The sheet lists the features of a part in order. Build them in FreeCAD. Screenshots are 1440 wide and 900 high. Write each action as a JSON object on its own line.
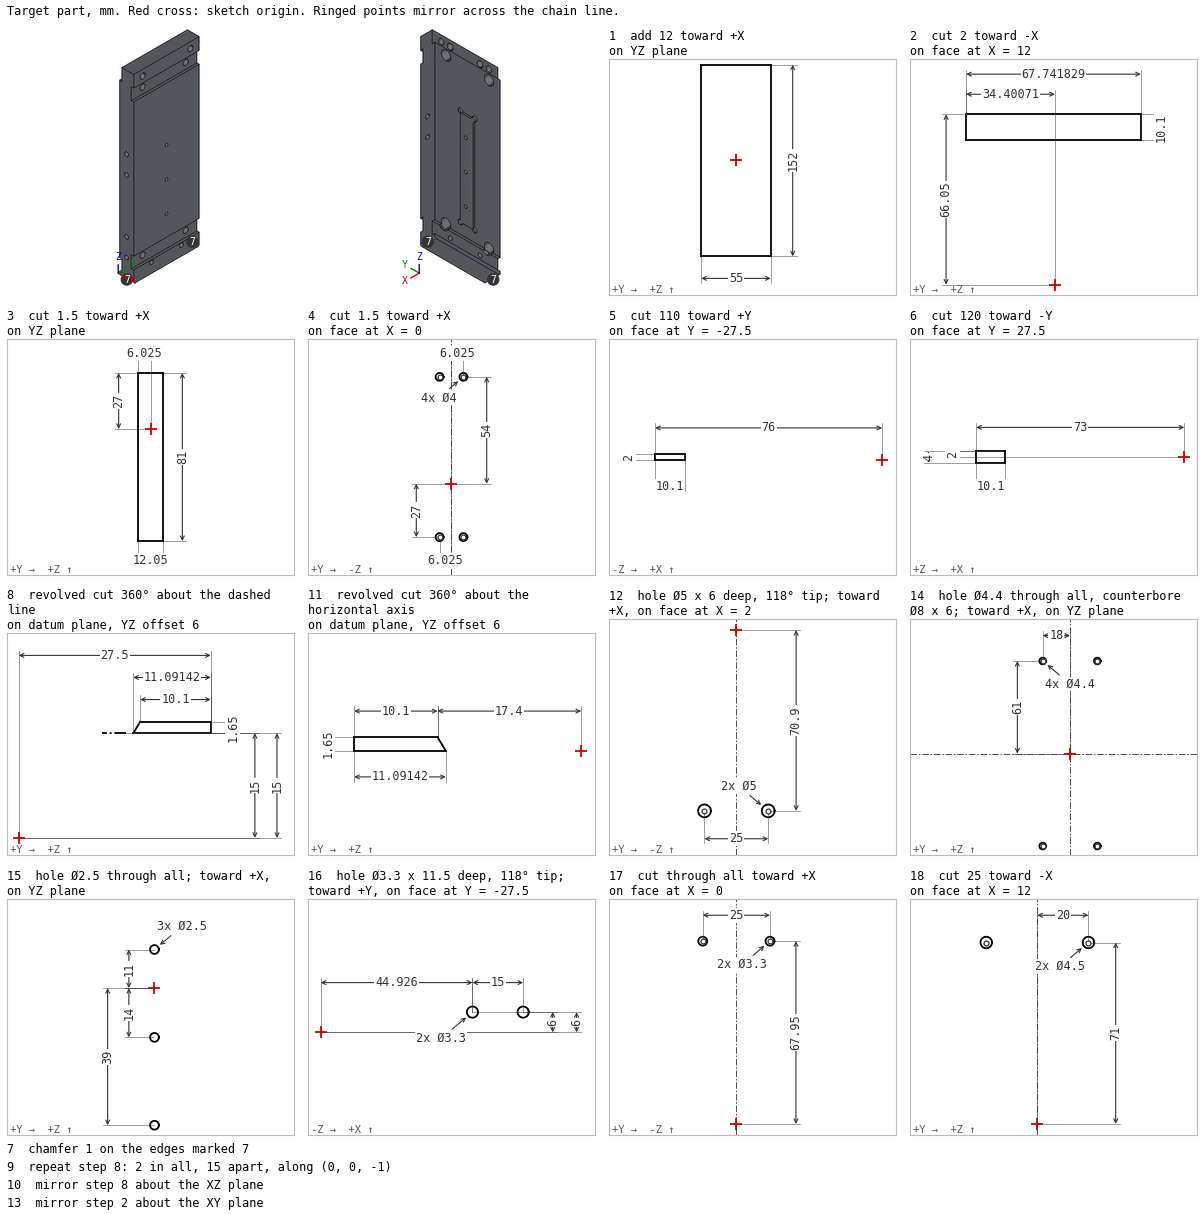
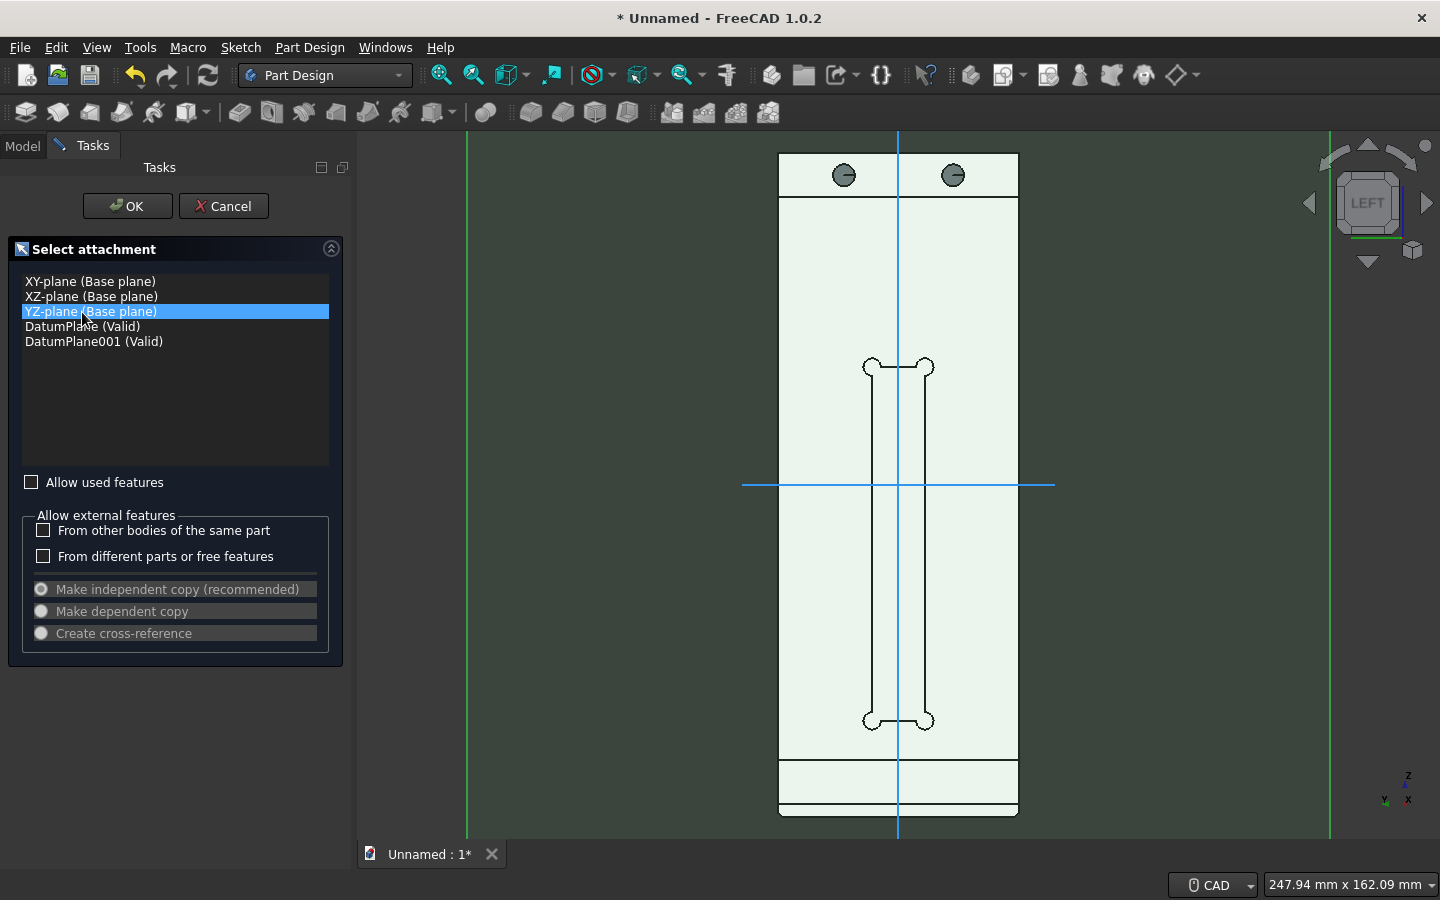
{"action": "left_click", "coordinate": [128, 206]}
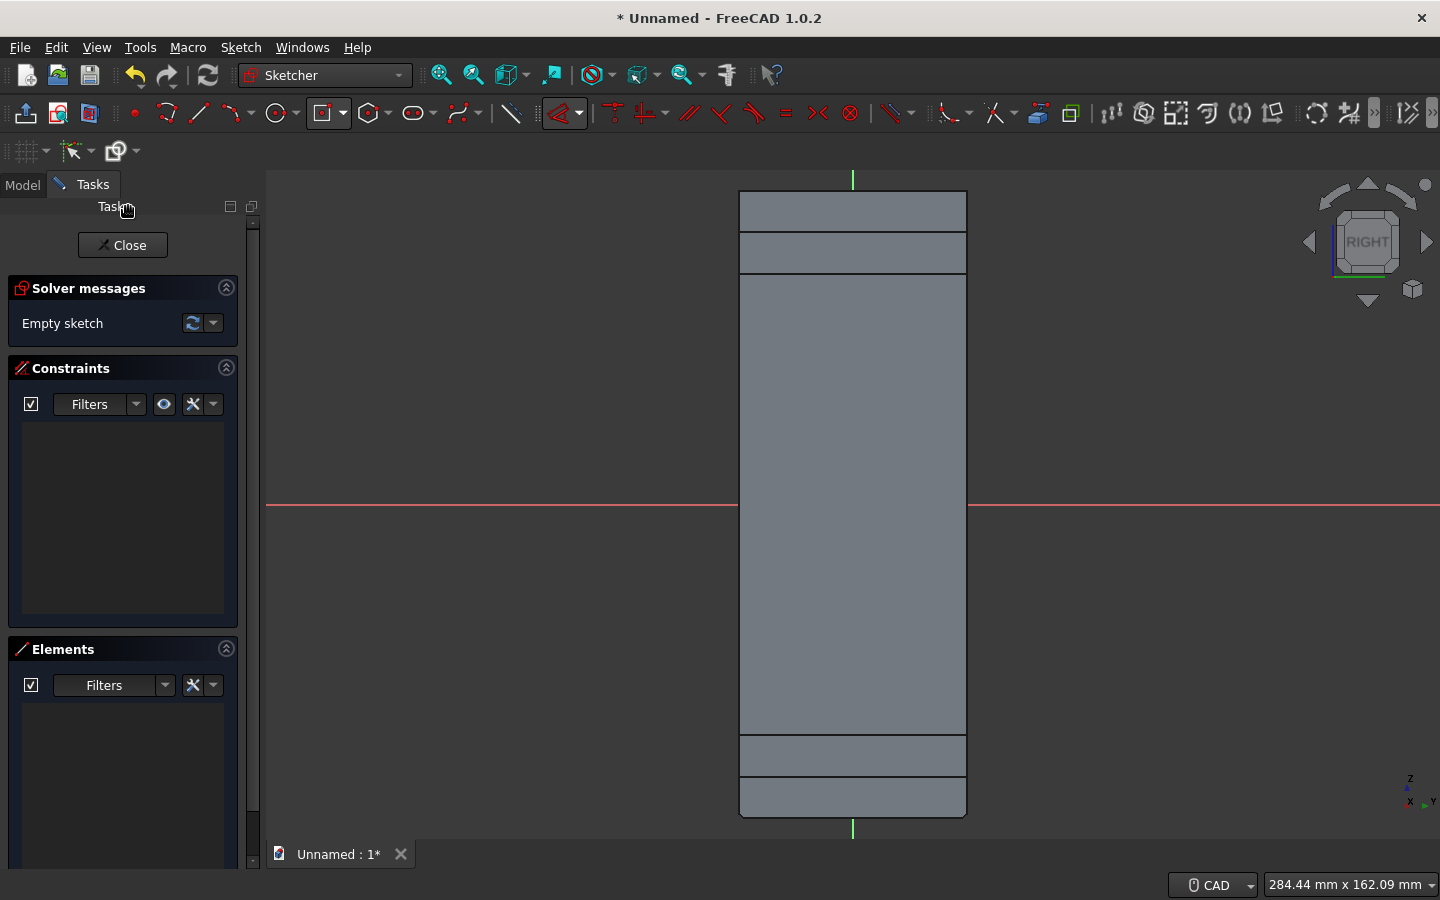
{"action": "key", "text": "q s"}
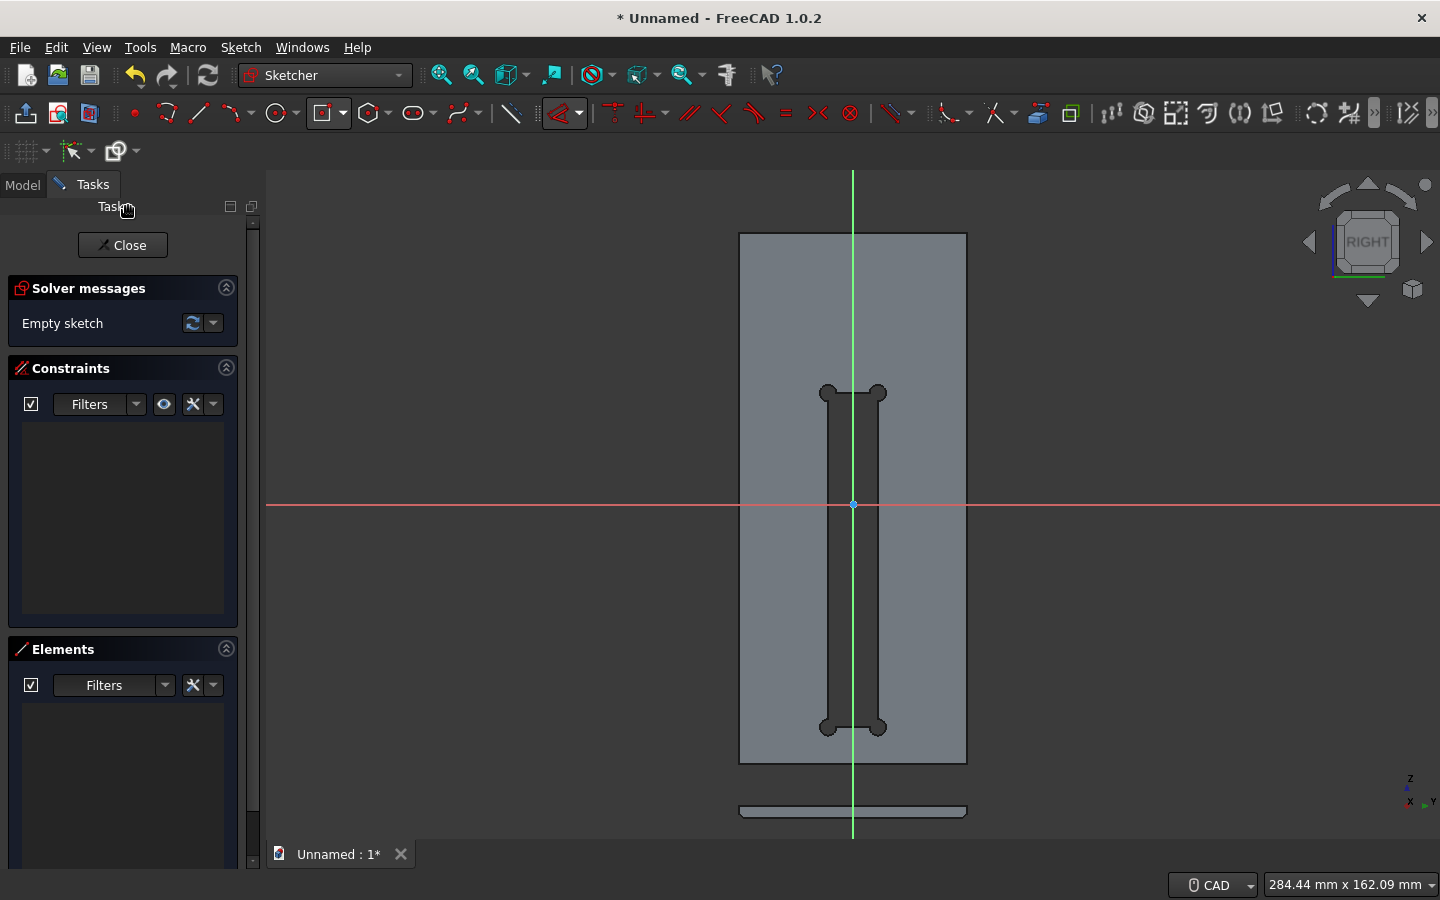
{"action": "left_click", "coordinate": [276, 114]}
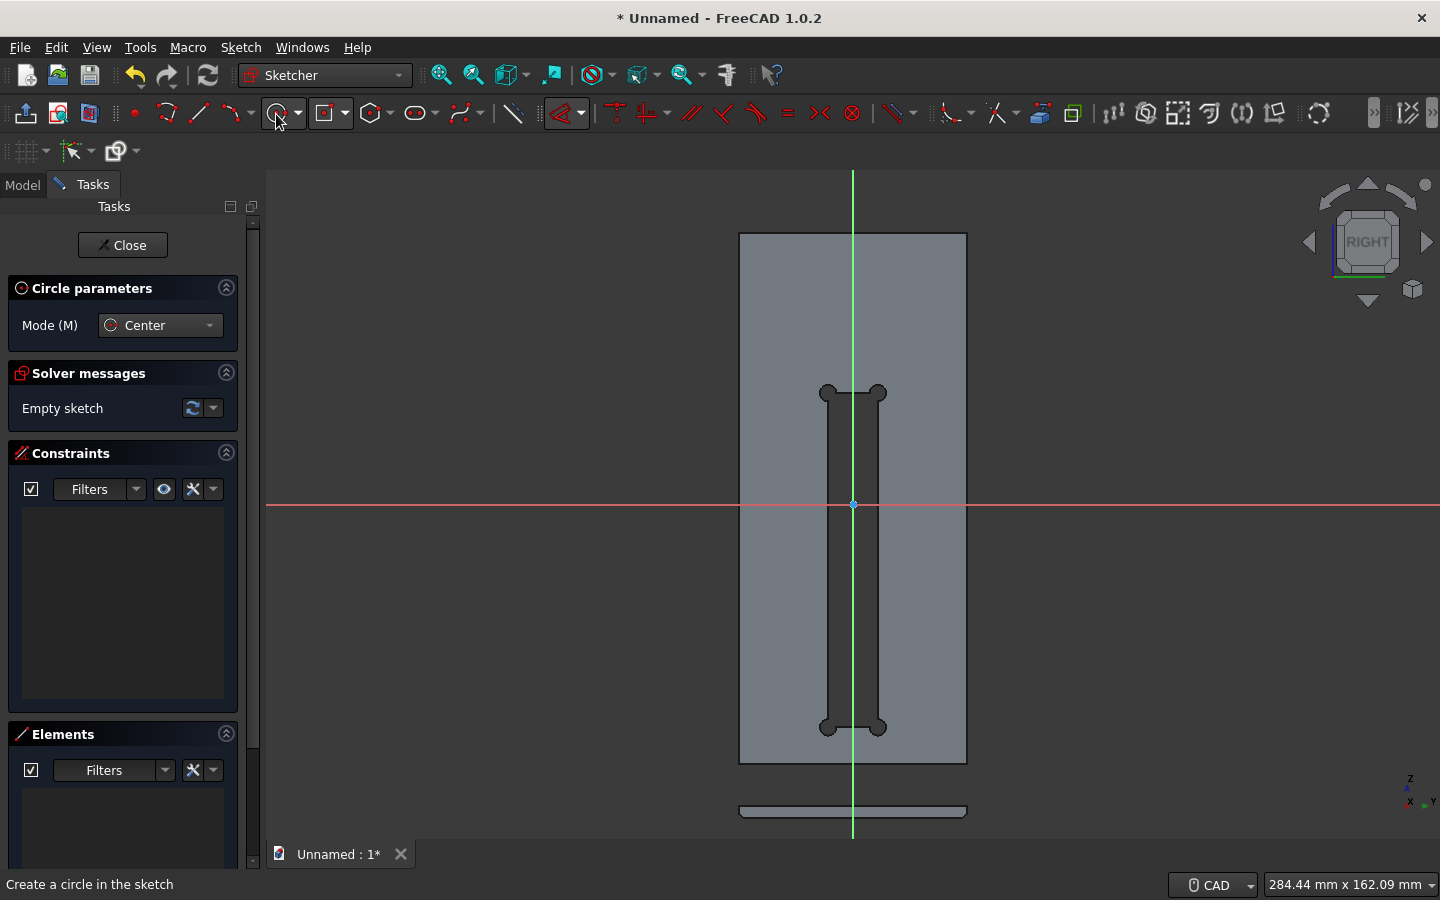
{"action": "scroll", "coordinate": [779, 253], "scroll_direction": "up", "scroll_amount": 5}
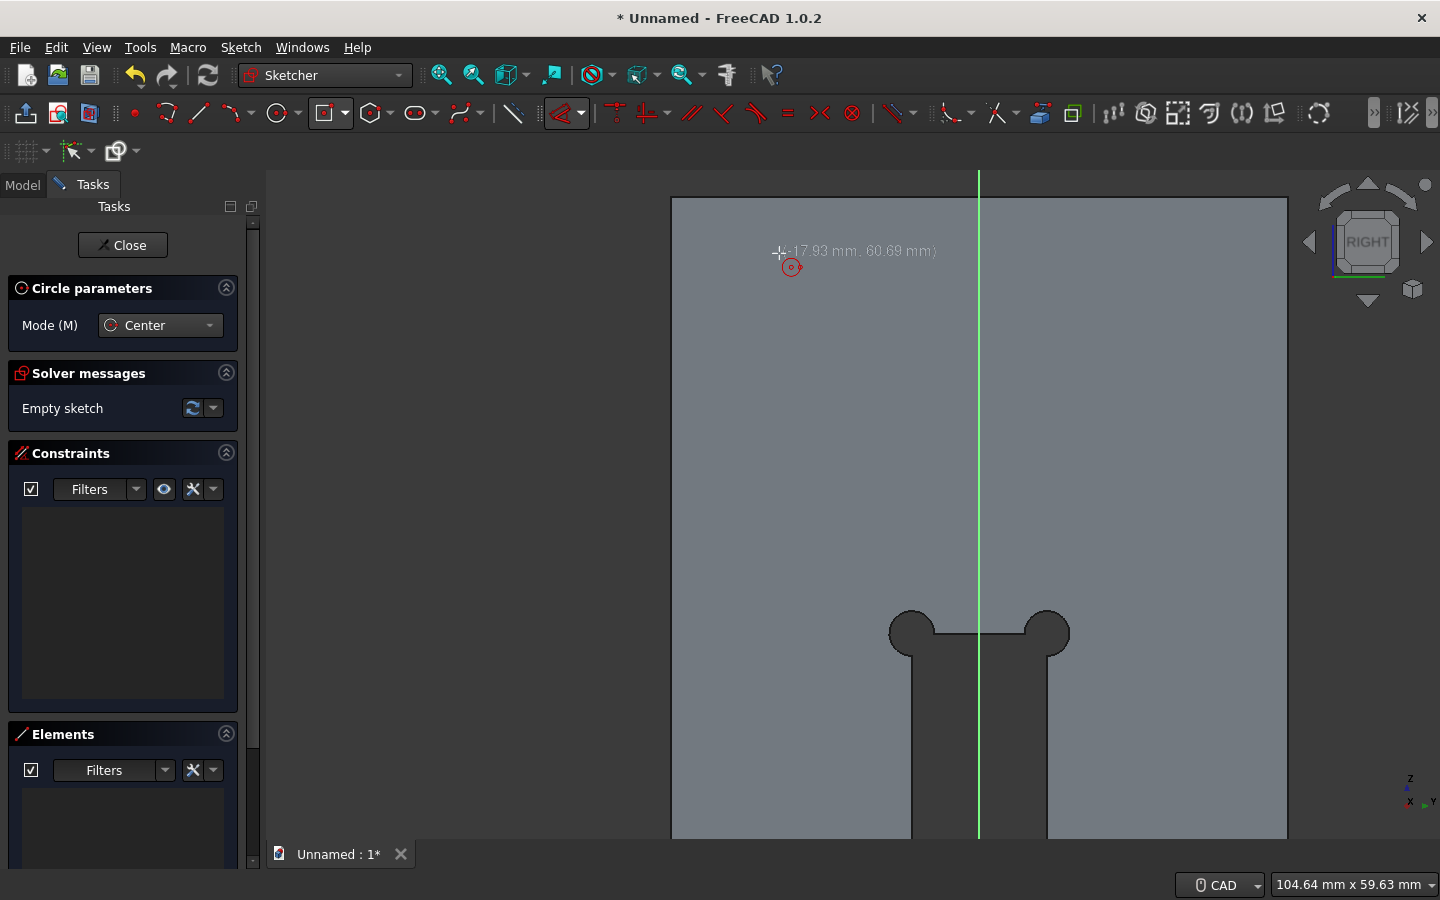
{"action": "left_click", "coordinate": [777, 252]}
{"action": "mouse_move", "coordinate": [795, 235]}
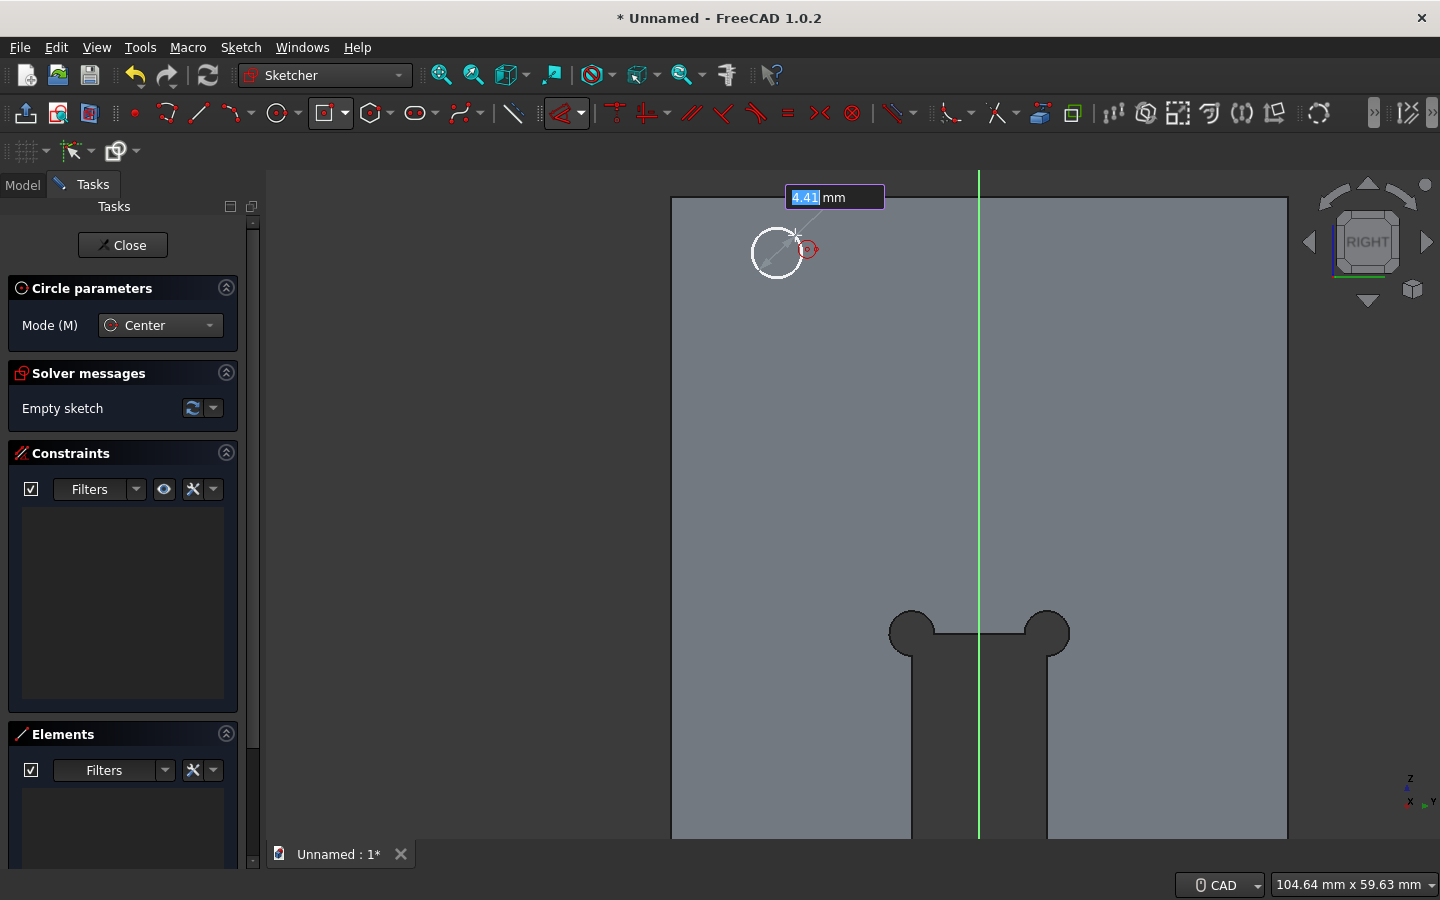
{"action": "type", "text": "4.4"}
{"action": "key", "text": "Return"}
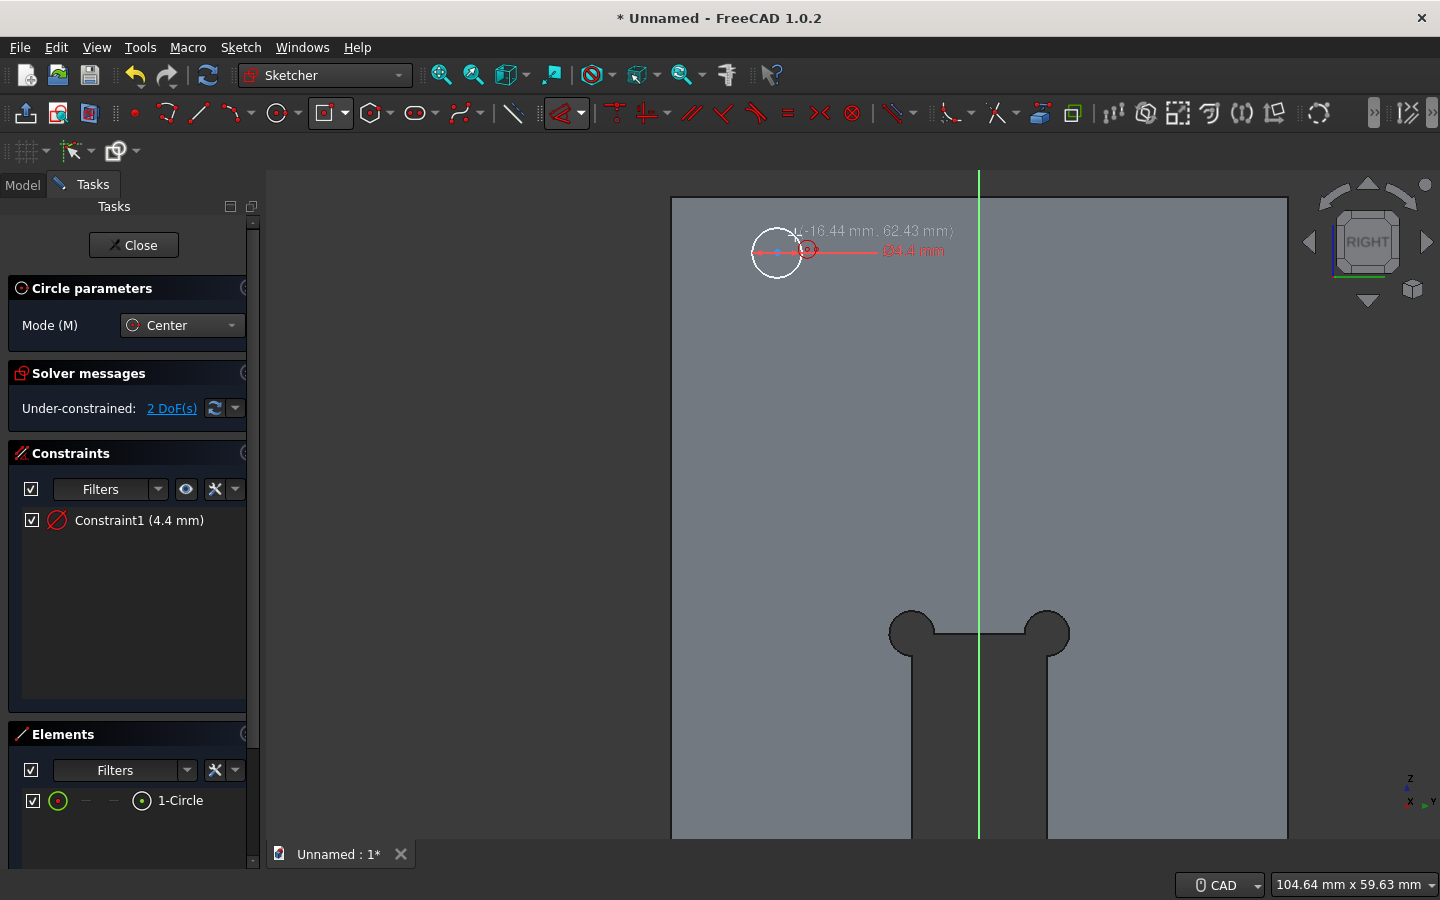
{"action": "left_click", "coordinate": [1181, 252]}
{"action": "mouse_move", "coordinate": [1199, 235]}